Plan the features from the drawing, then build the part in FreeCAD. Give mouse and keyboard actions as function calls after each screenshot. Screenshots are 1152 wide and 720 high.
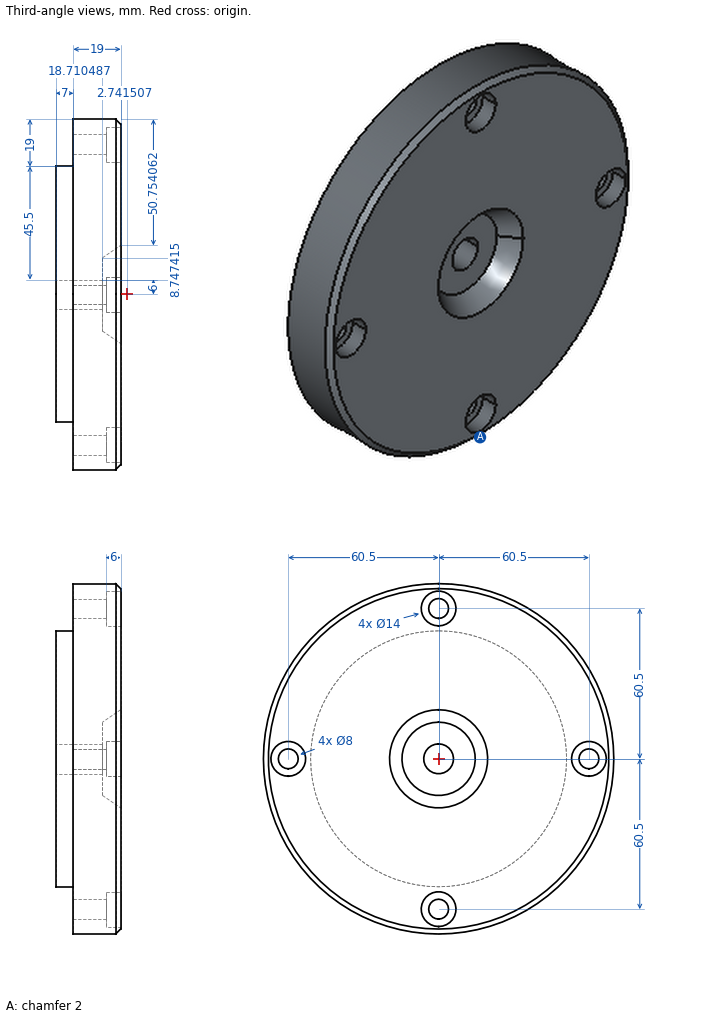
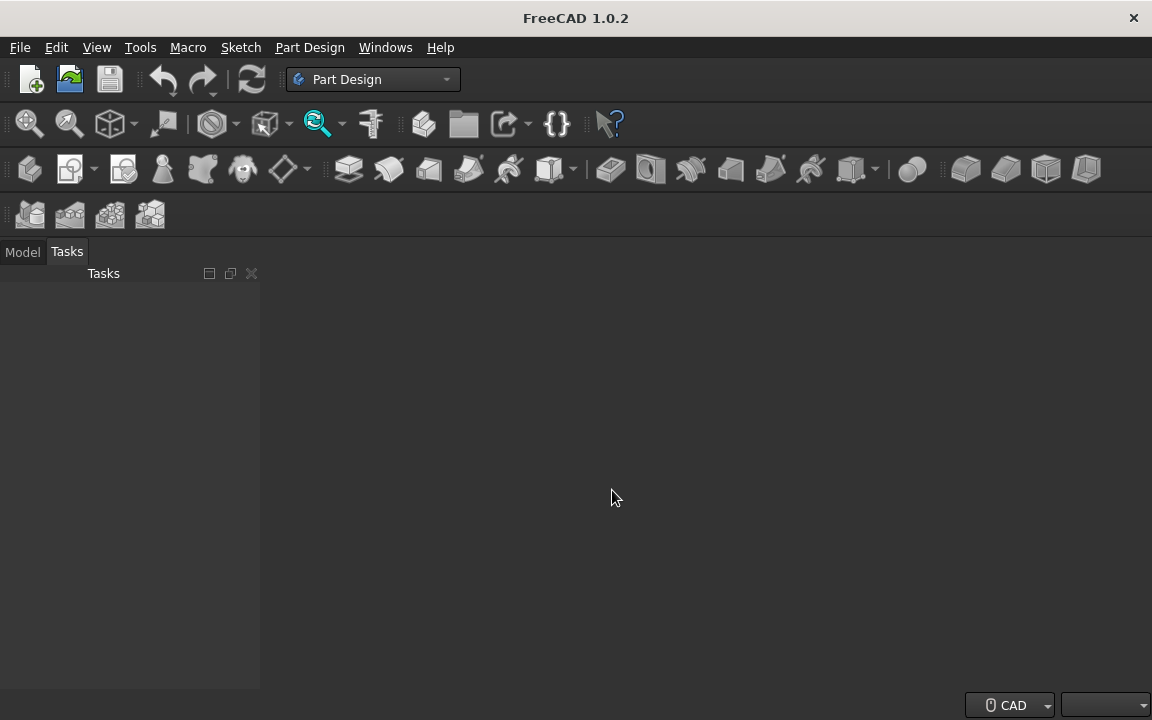
click(30, 80)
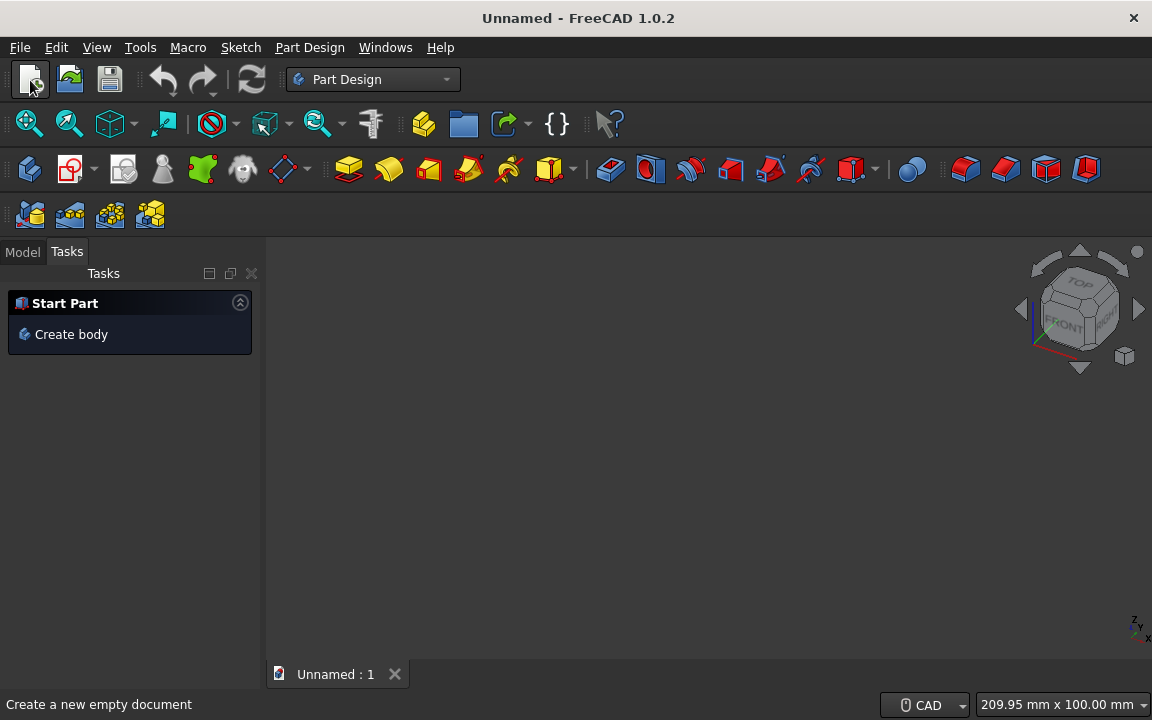
click(70, 170)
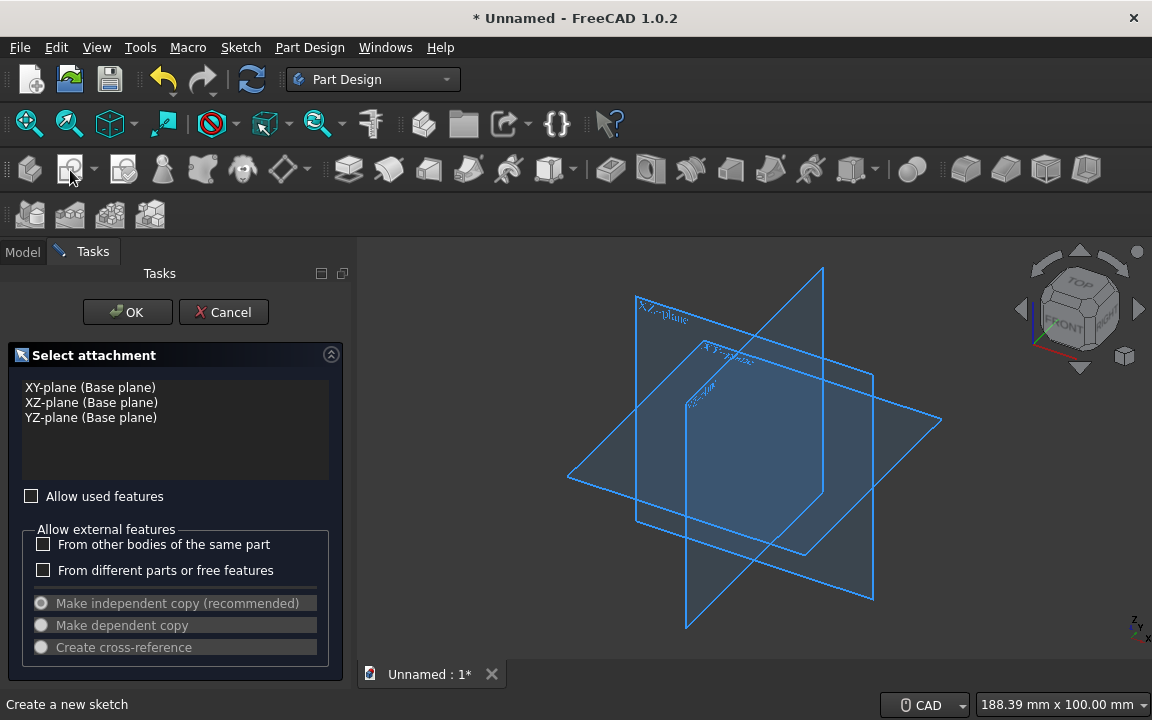
click(82, 388)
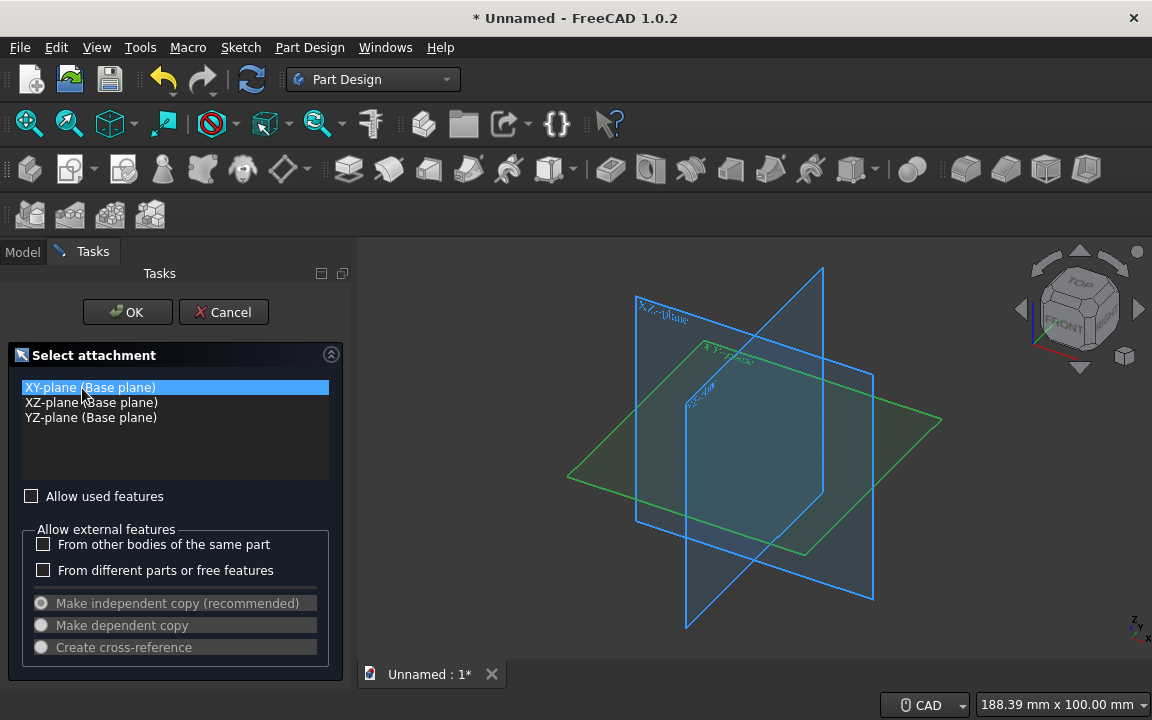
click(128, 312)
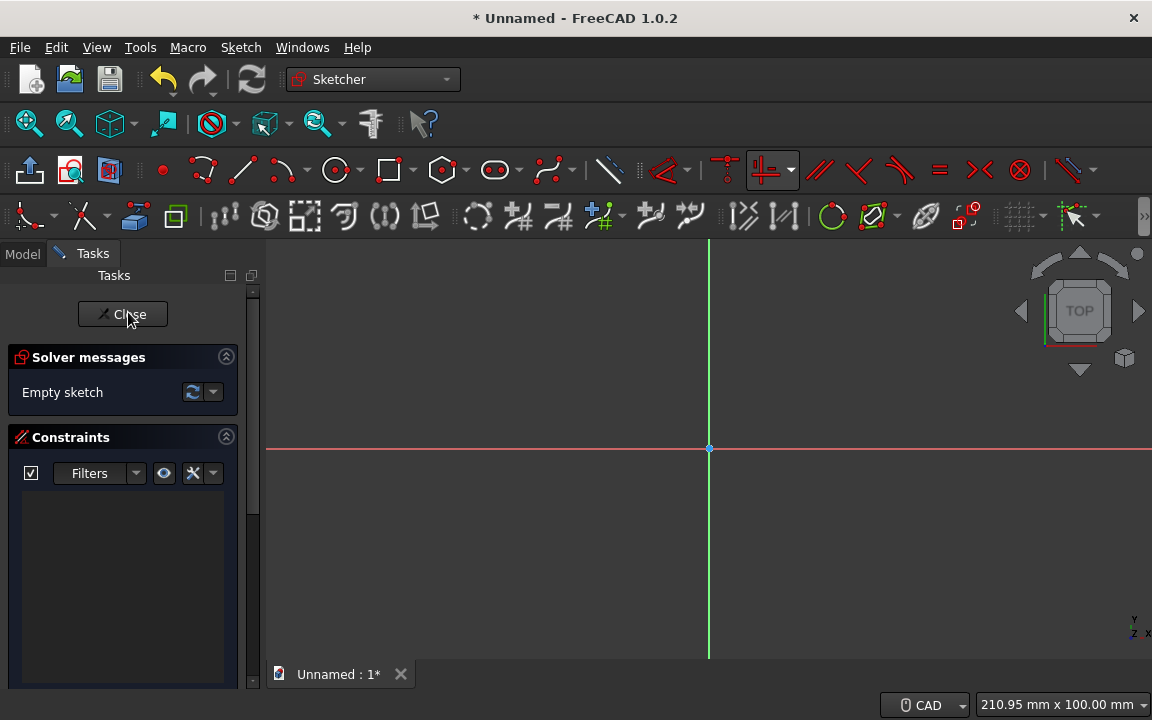
scroll(624, 631, down, 2)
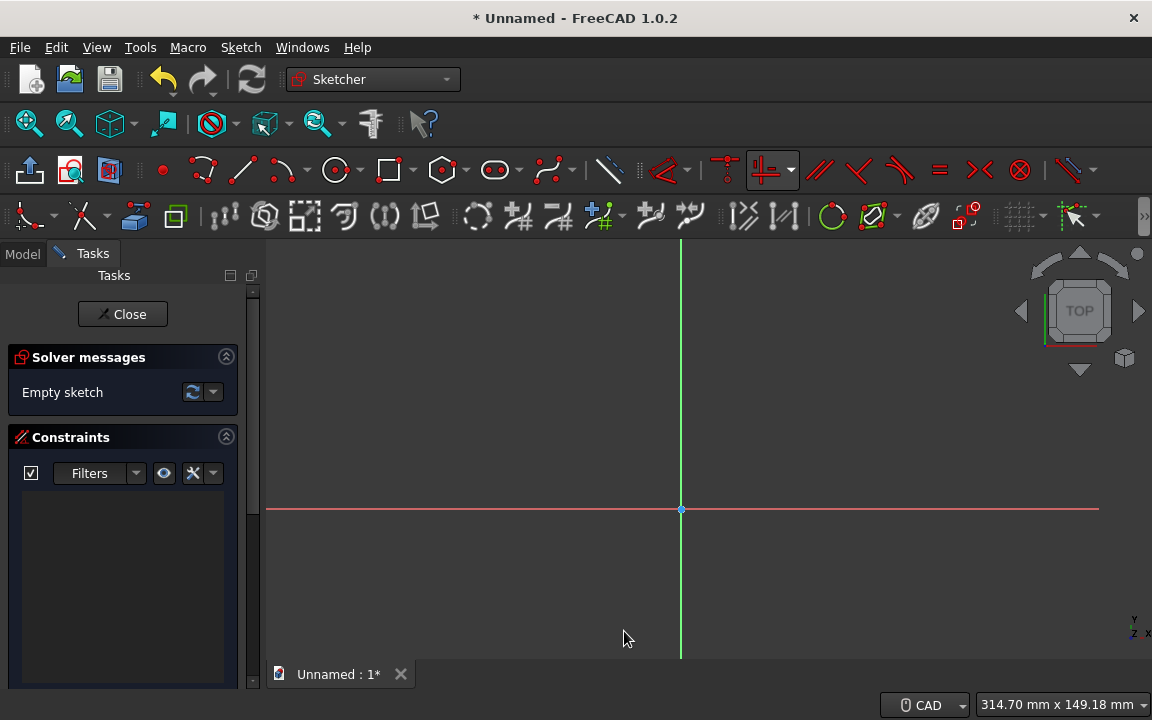
click(204, 170)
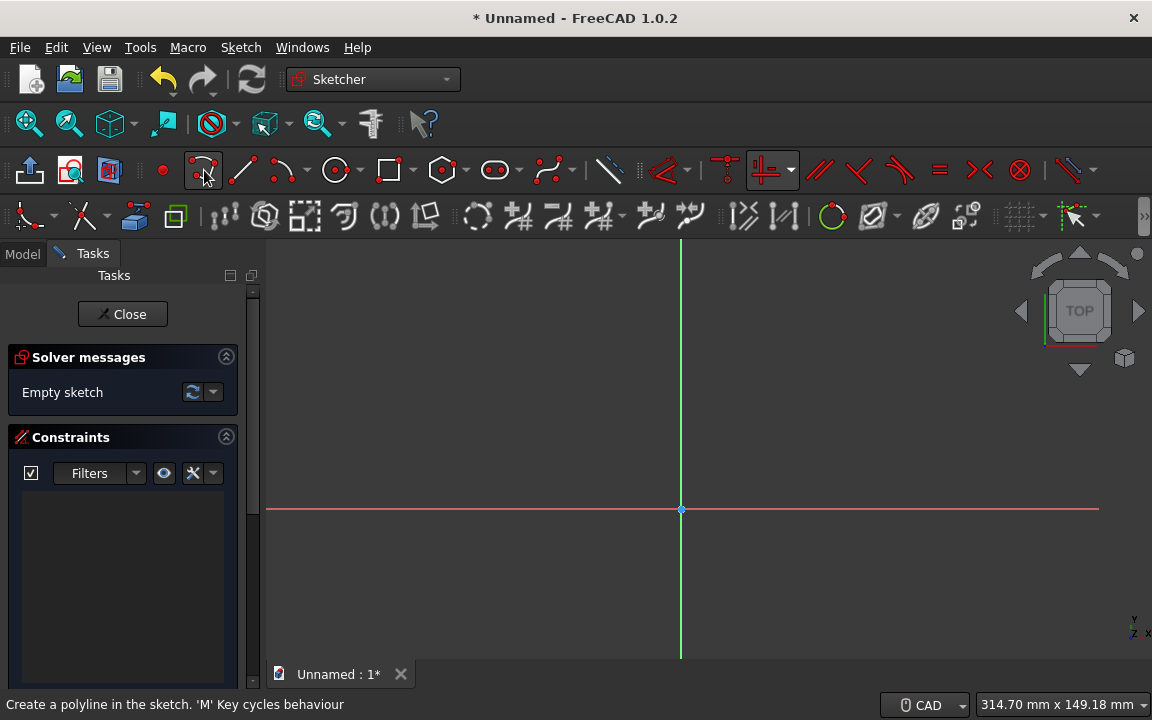
click(653, 492)
click(653, 468)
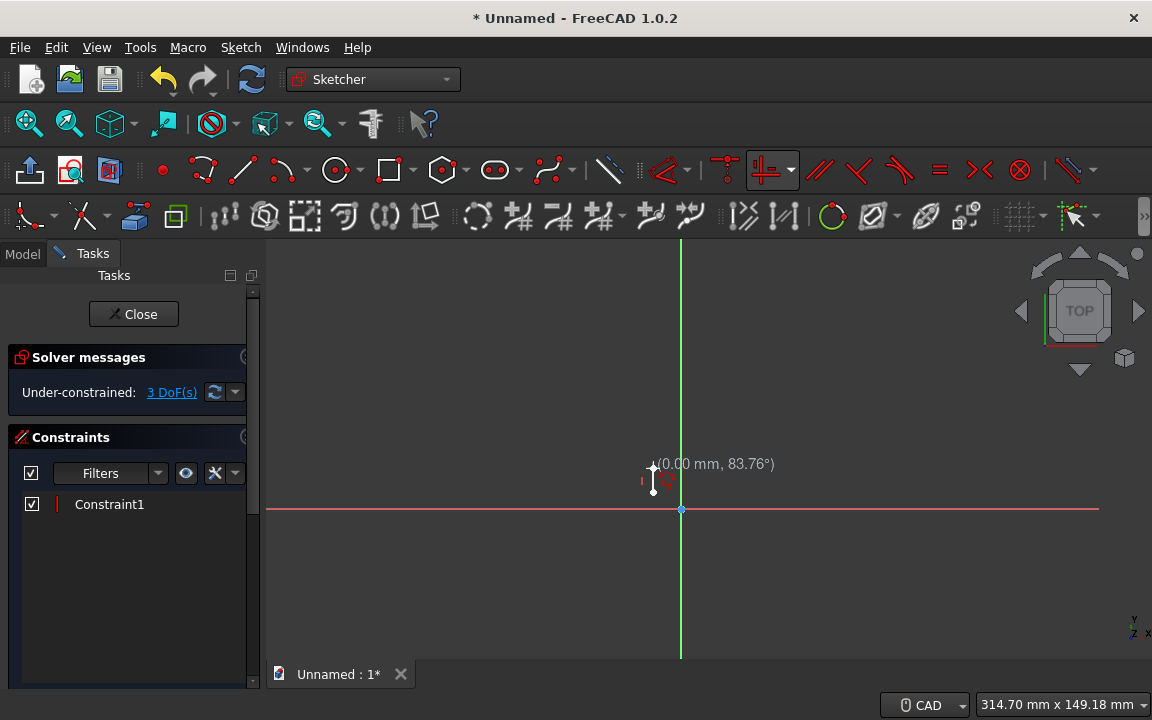
scroll(673, 454, up, 4)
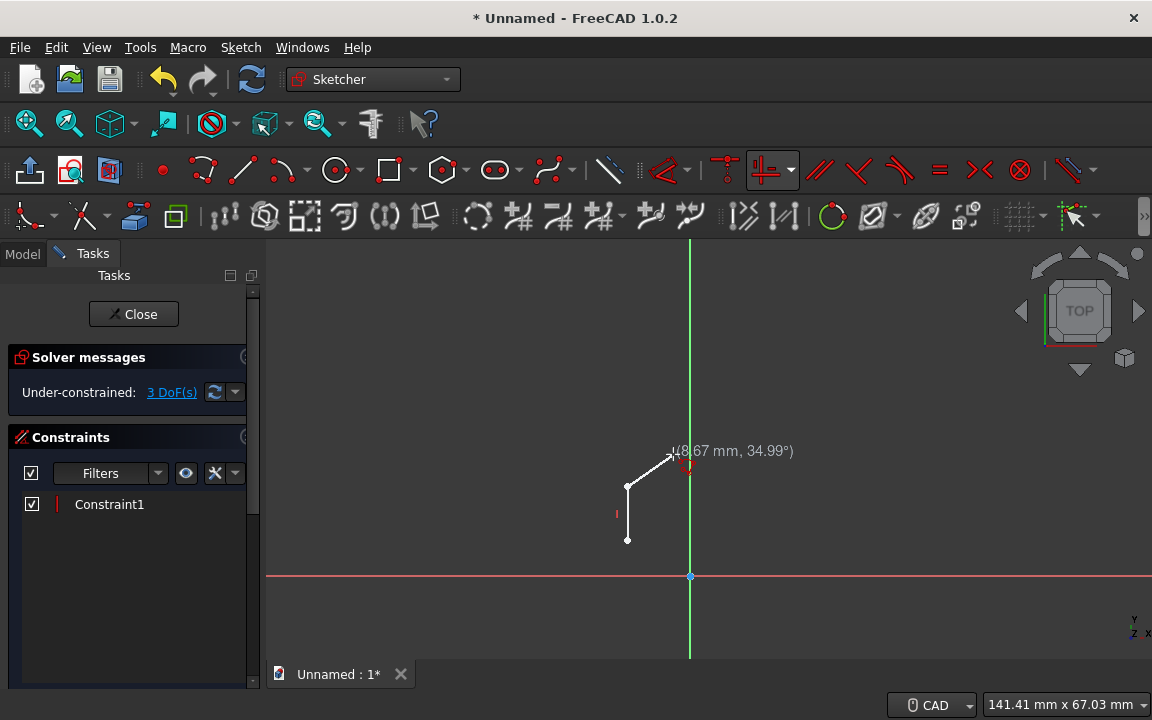
click(673, 453)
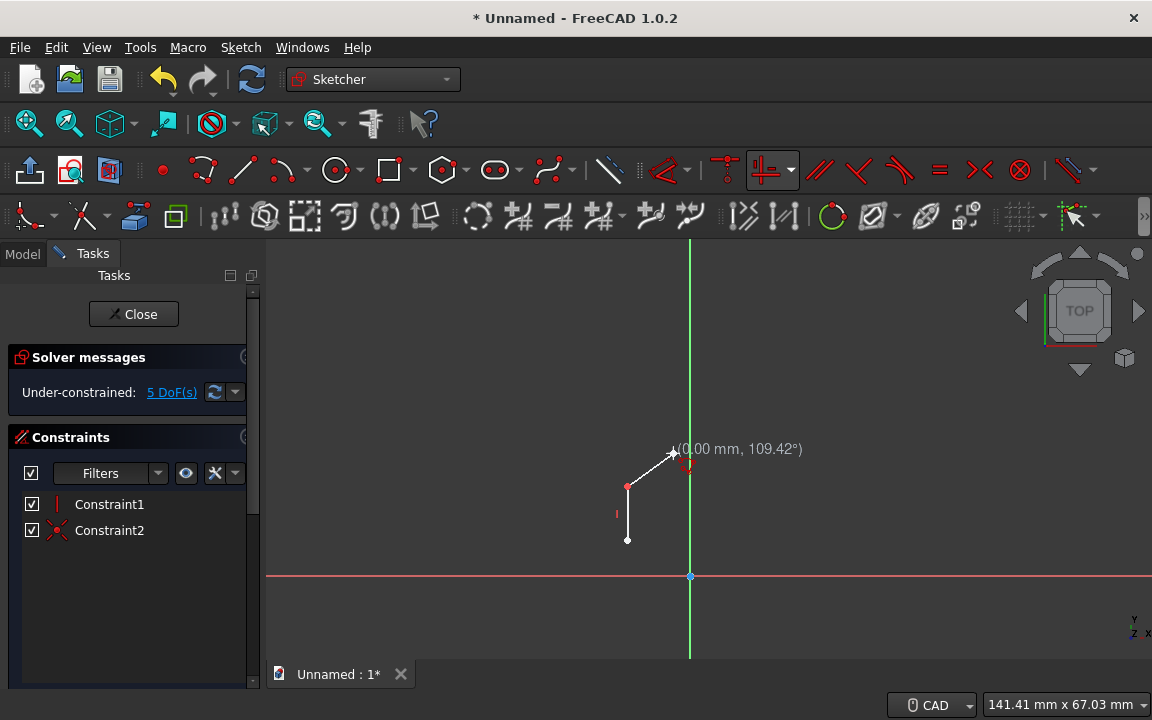
scroll(689, 563, down, 3)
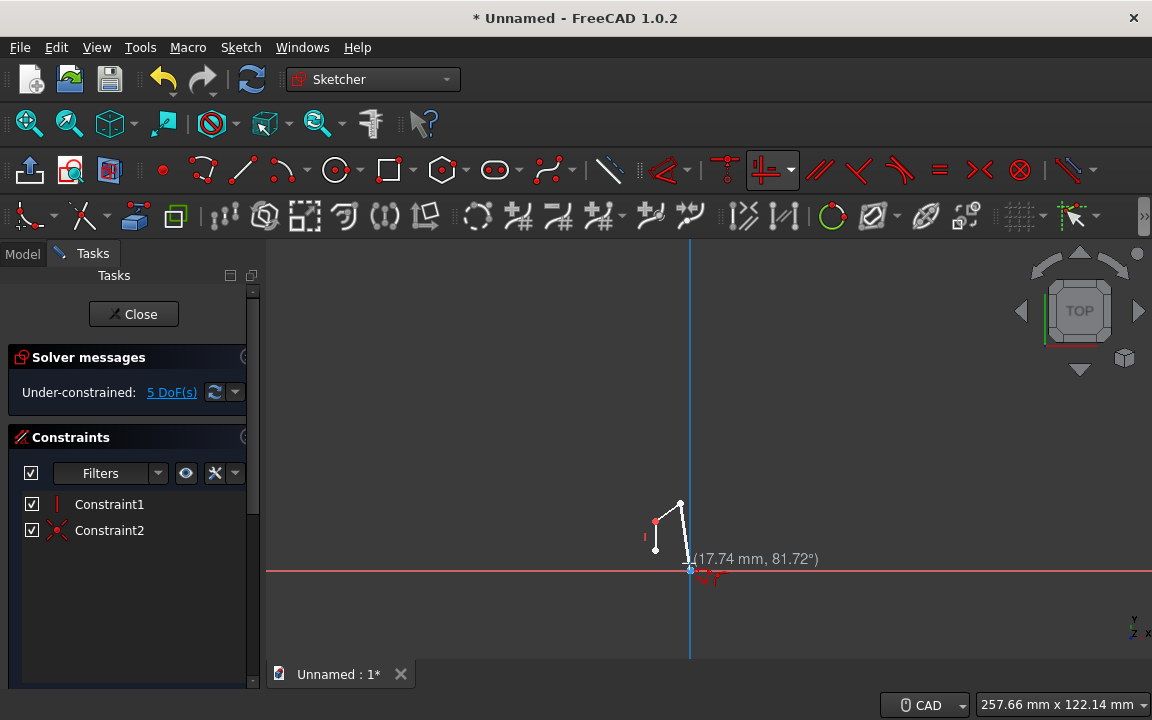
scroll(681, 328, up, 3)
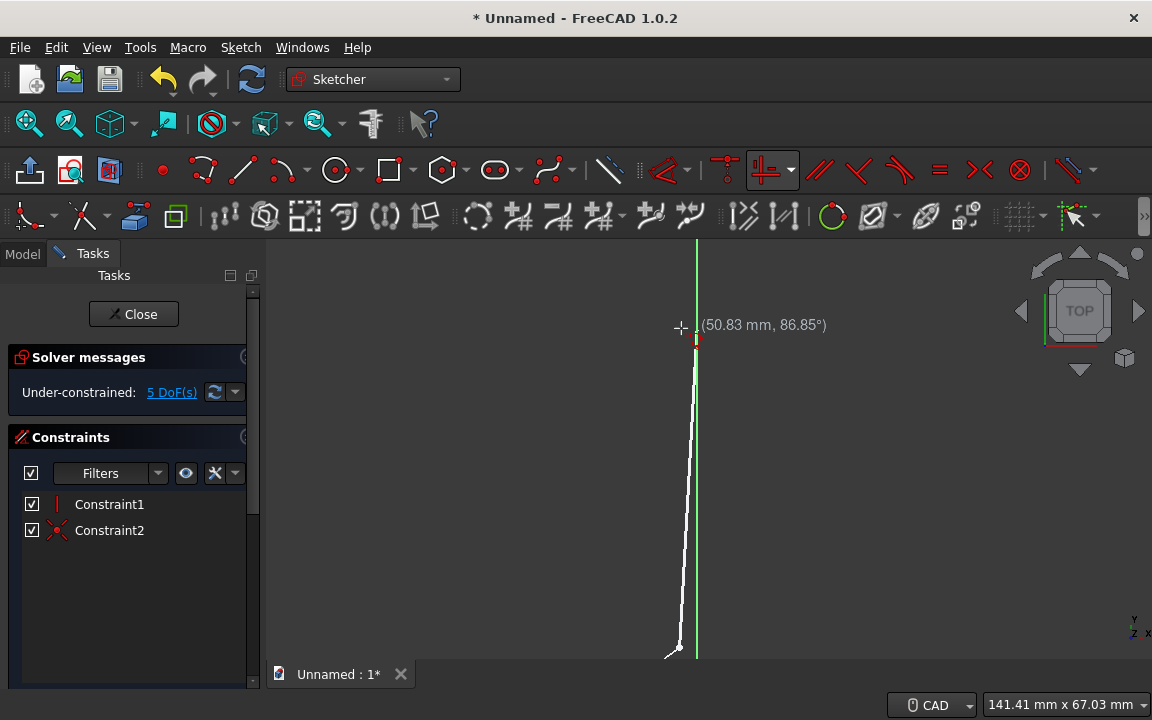
click(680, 328)
click(561, 328)
click(561, 447)
click(517, 447)